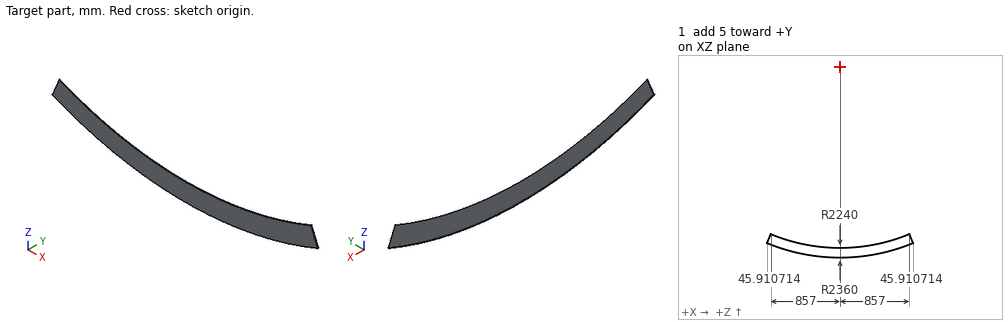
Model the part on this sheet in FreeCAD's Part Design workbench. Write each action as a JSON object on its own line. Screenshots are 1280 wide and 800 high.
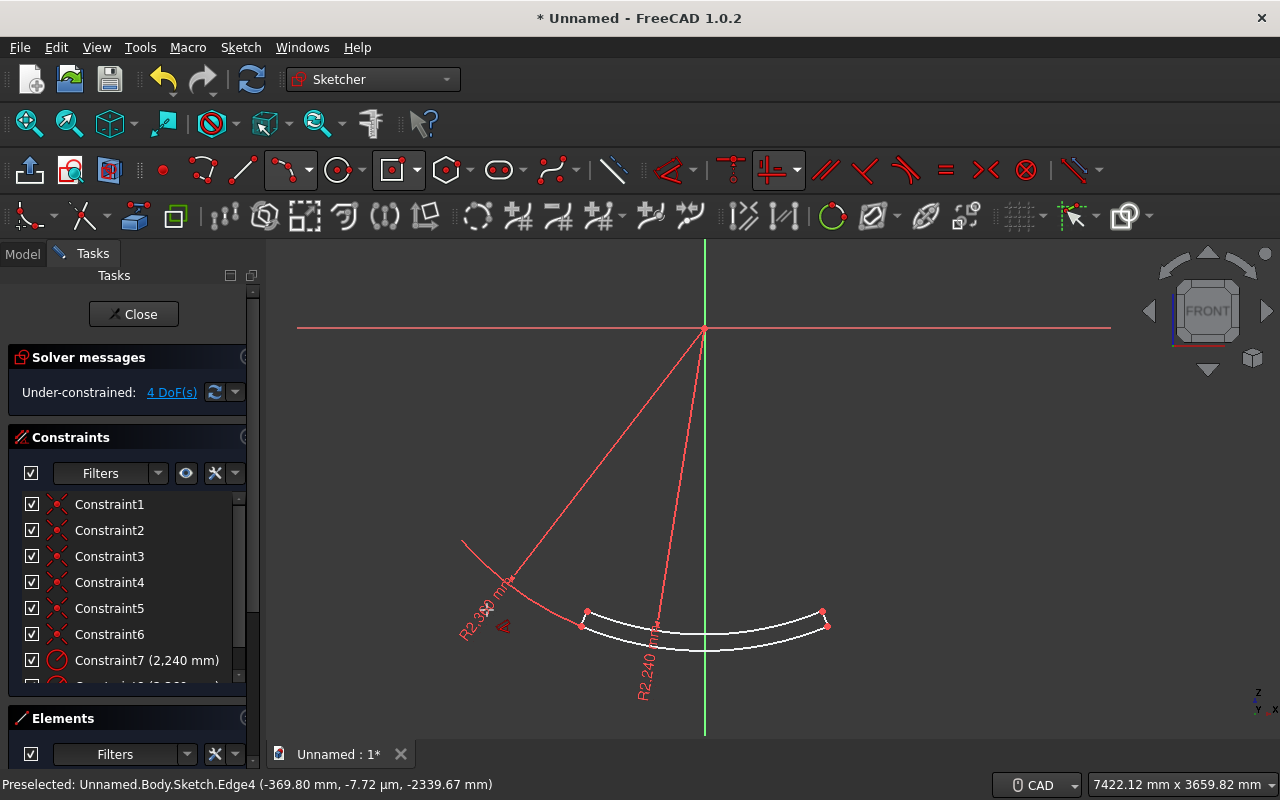
{"action": "left_click", "coordinate": [587, 611]}
{"action": "left_click", "coordinate": [646, 294]}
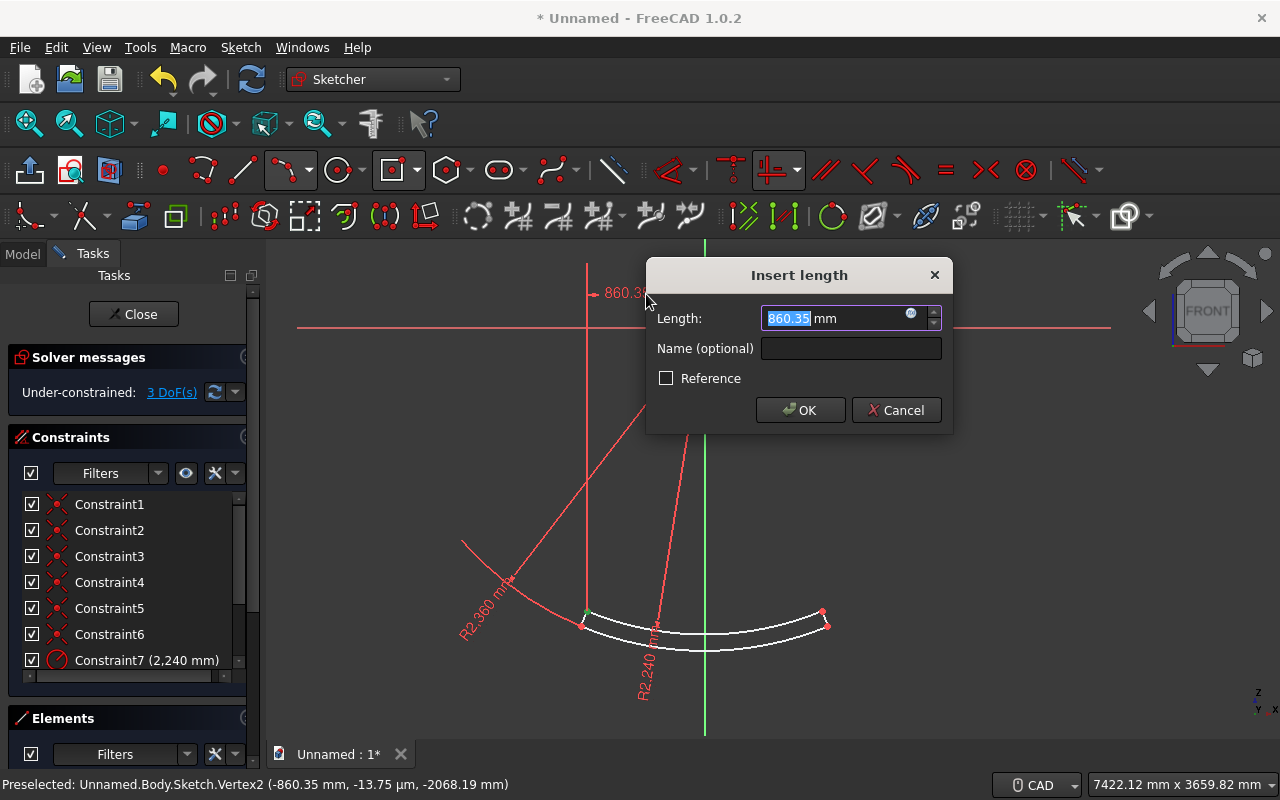
{"action": "type", "text": "857"}
{"action": "key", "text": "Return"}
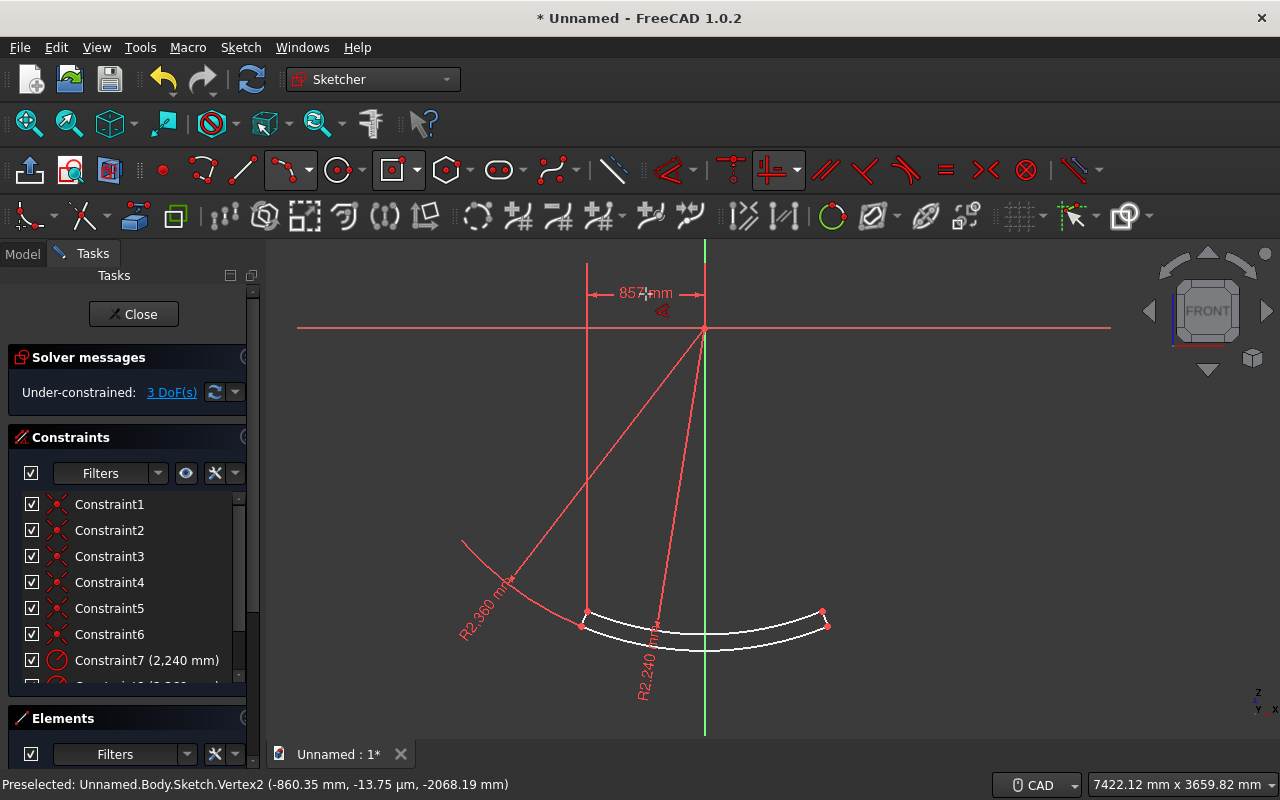
{"action": "left_click", "coordinate": [822, 611]}
{"action": "left_click", "coordinate": [763, 294]}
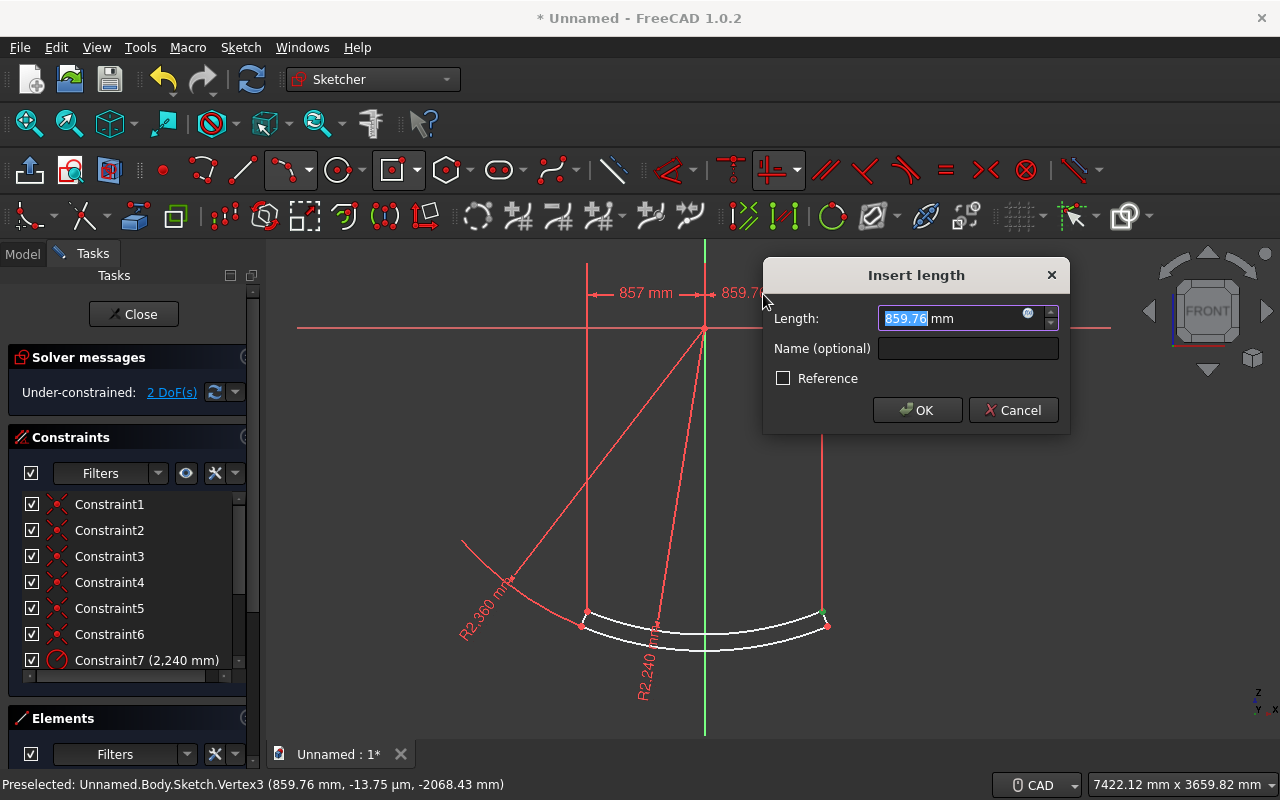
{"action": "type", "text": "857"}
{"action": "key", "text": "Return"}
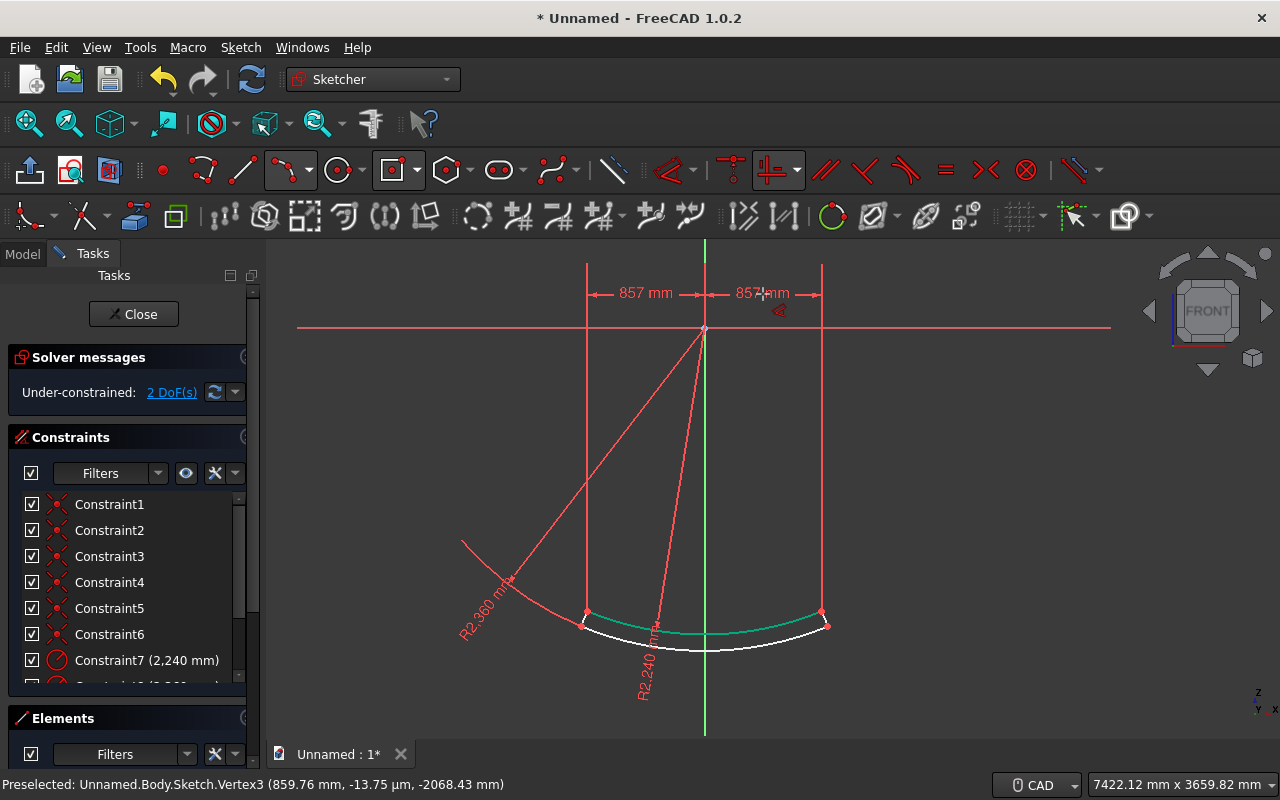
{"action": "scroll", "coordinate": [584, 619], "scroll_direction": "up", "scroll_amount": 10}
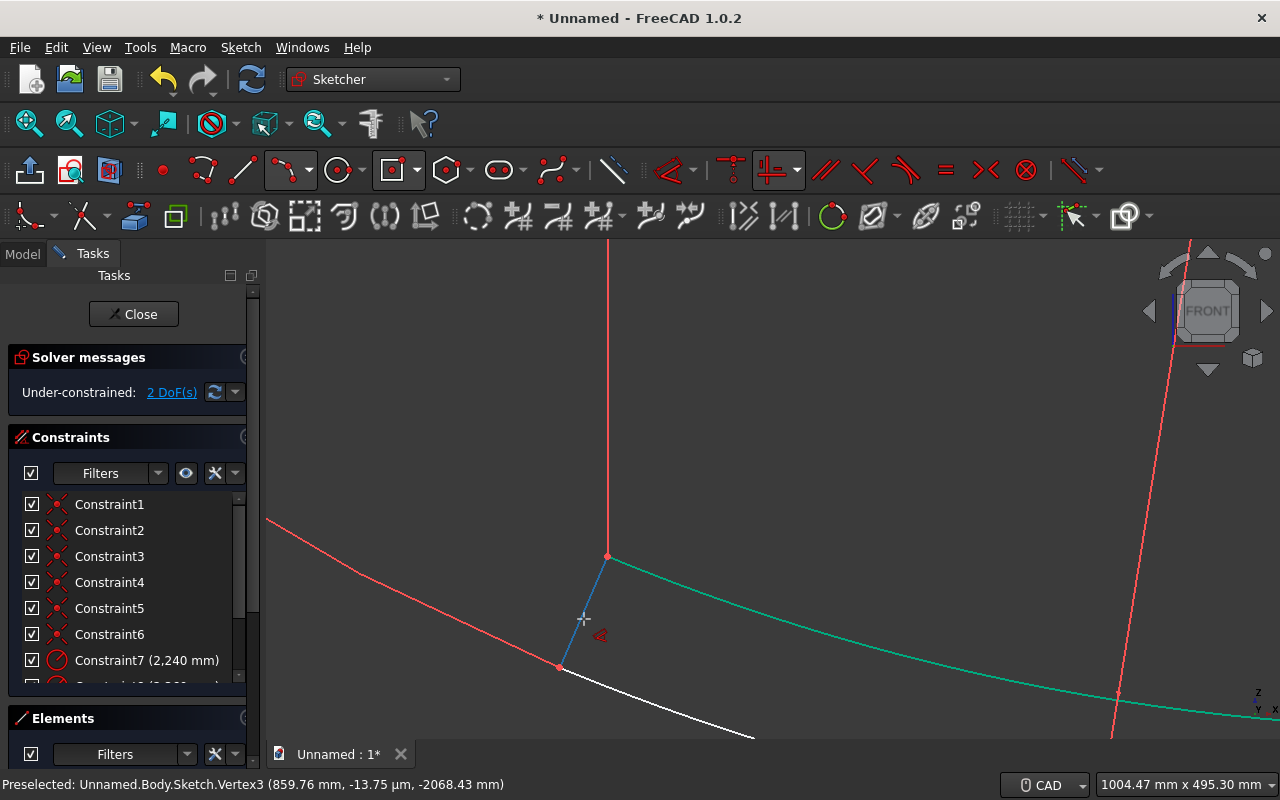
{"action": "left_click", "coordinate": [584, 612]}
{"action": "left_click", "coordinate": [584, 702]}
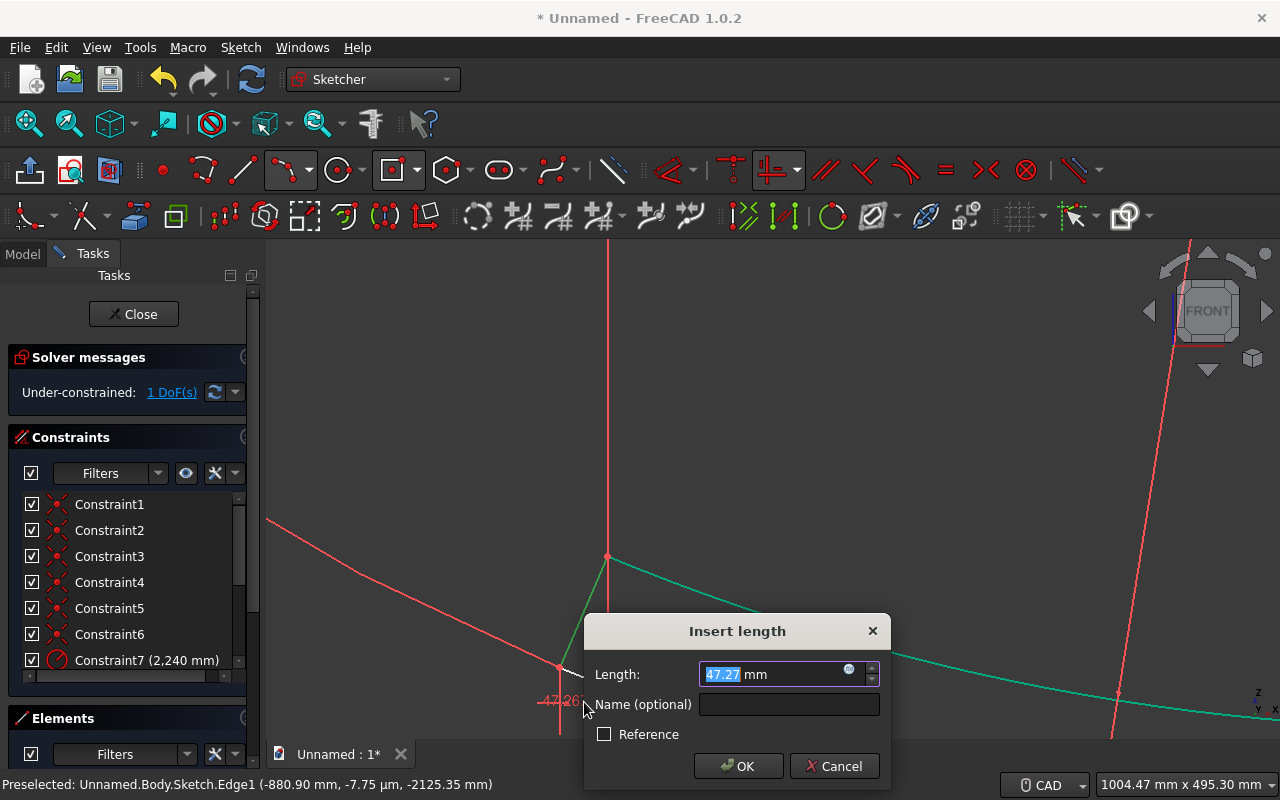
{"action": "type", "text": "45.910714"}
{"action": "key", "text": "Return"}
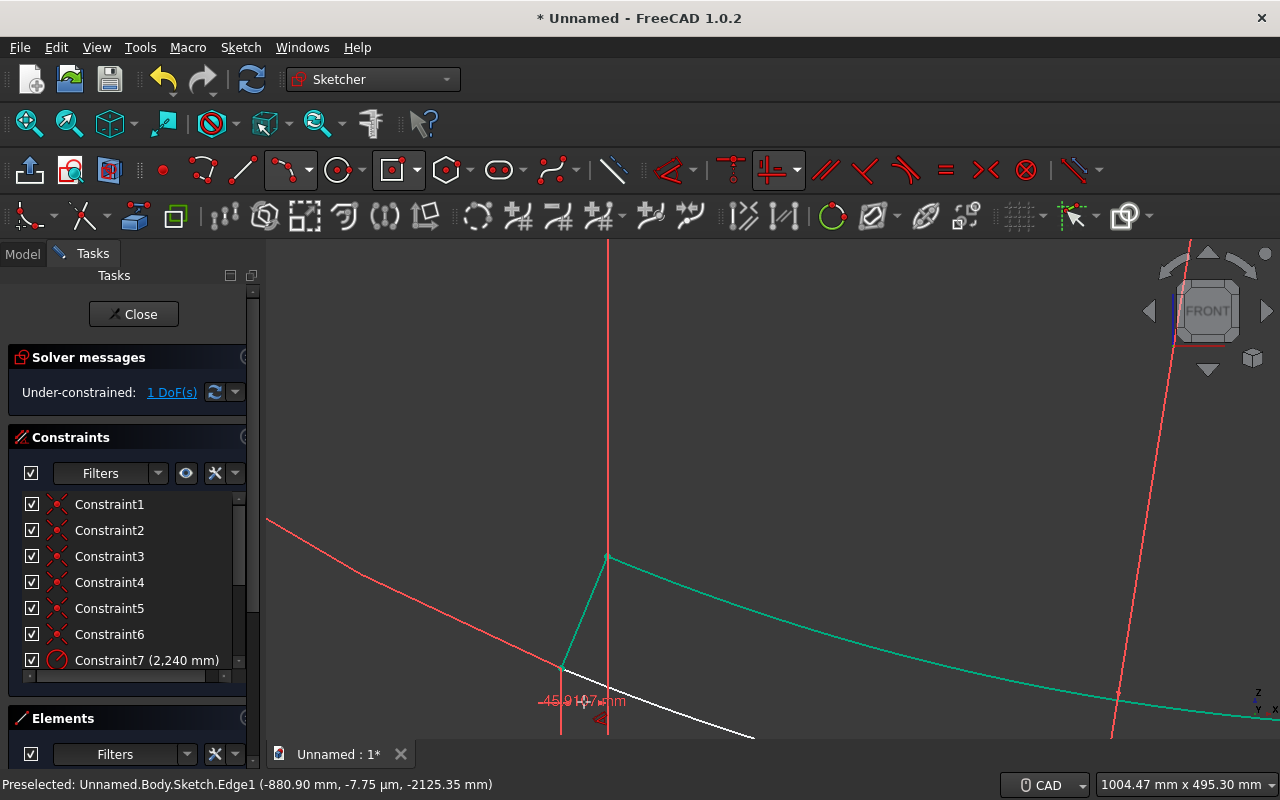
{"action": "scroll", "coordinate": [584, 619], "scroll_direction": "down", "scroll_amount": 10}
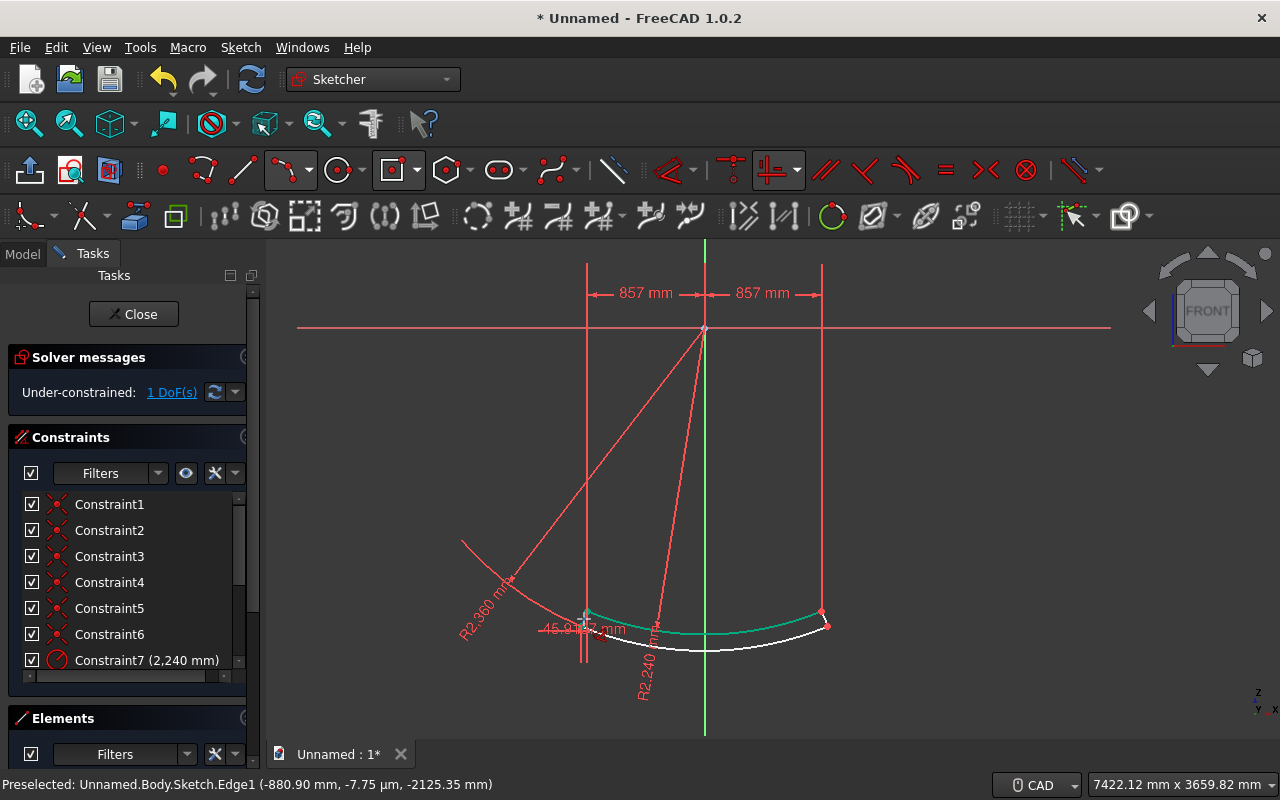
{"action": "scroll", "coordinate": [824, 616], "scroll_direction": "up", "scroll_amount": 10}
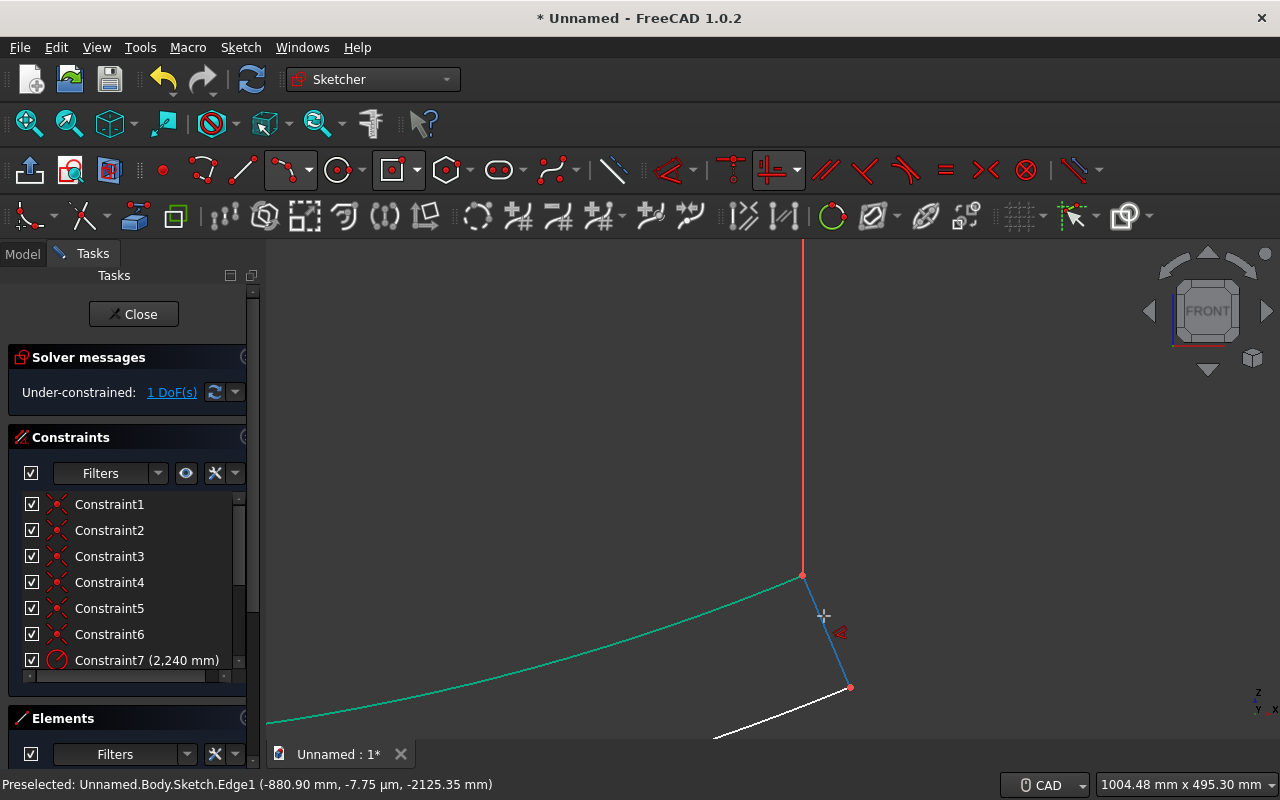
{"action": "left_click", "coordinate": [817, 609]}
{"action": "left_click", "coordinate": [826, 542]}